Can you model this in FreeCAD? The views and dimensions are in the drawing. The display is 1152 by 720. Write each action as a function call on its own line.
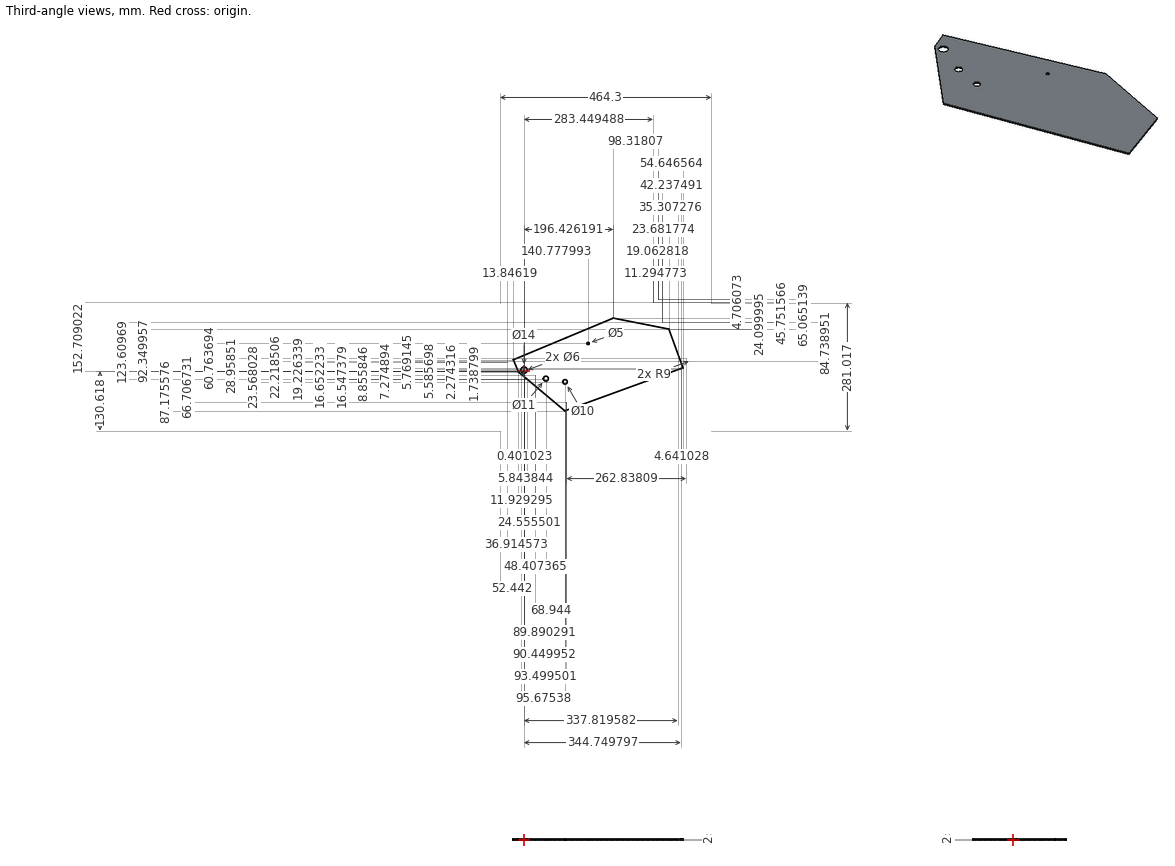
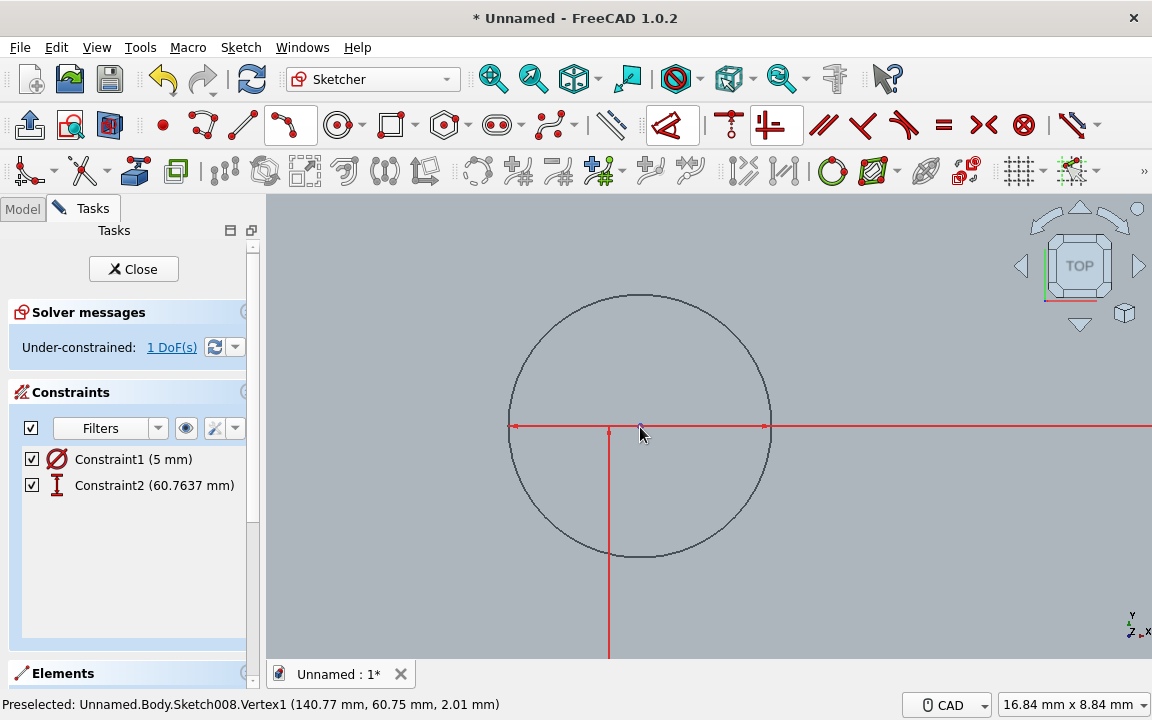
click(640, 426)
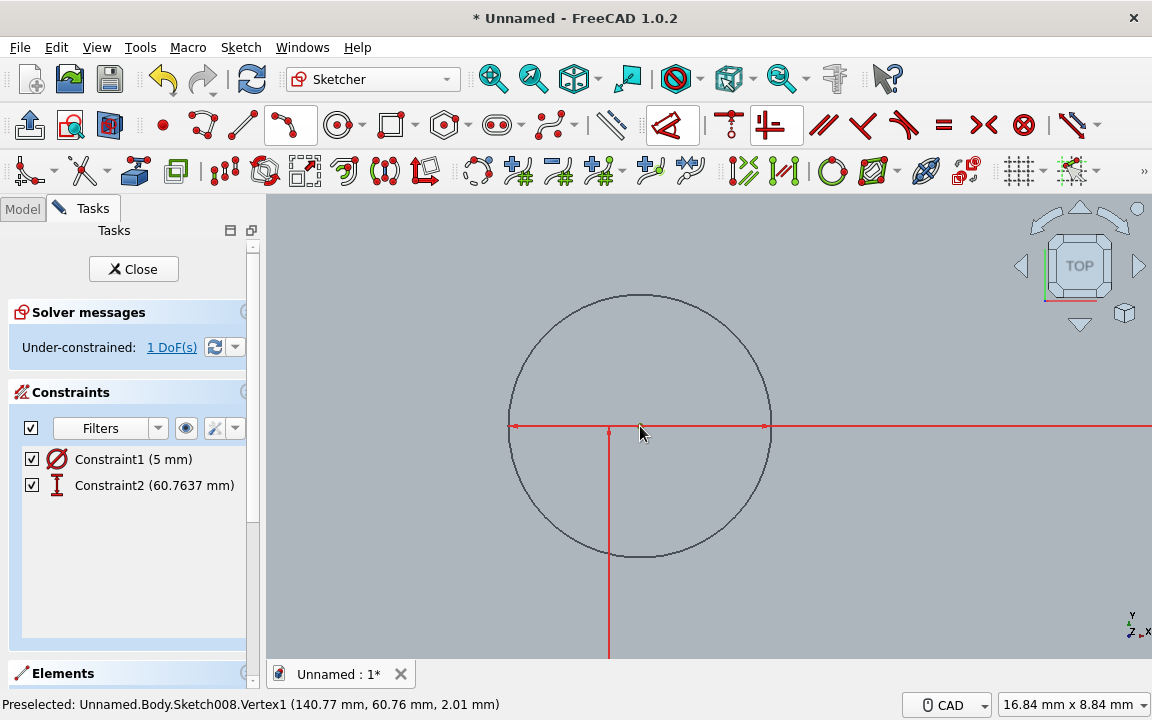
click(694, 126)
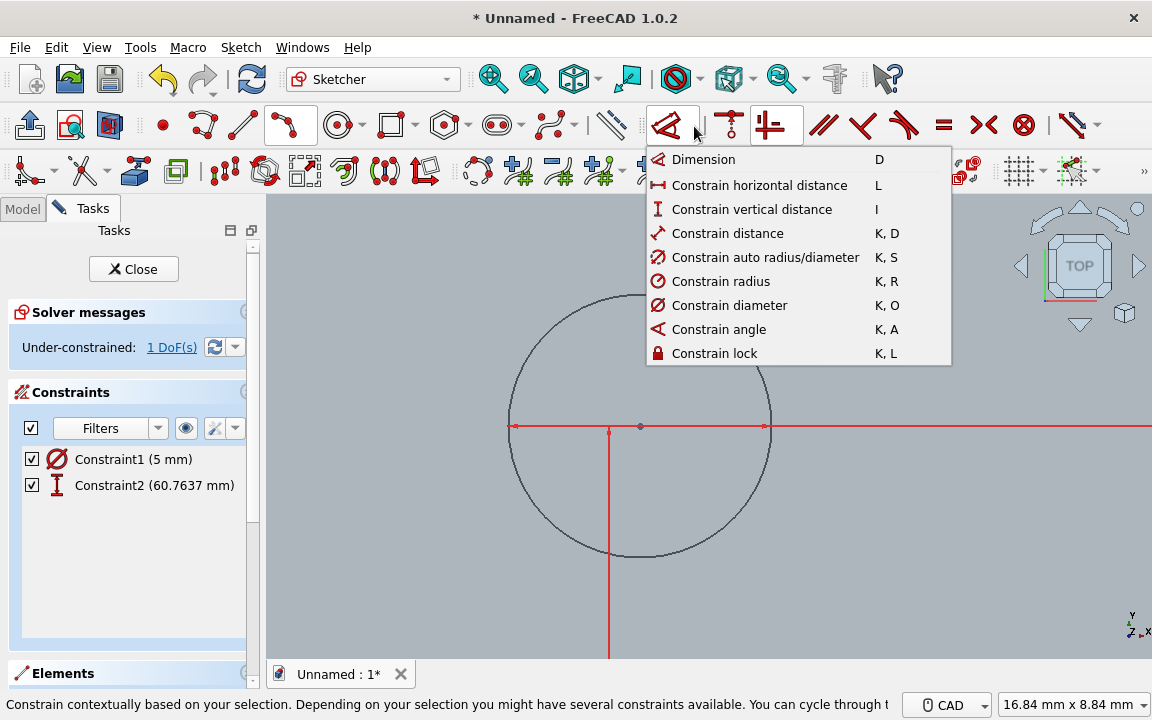
click(799, 185)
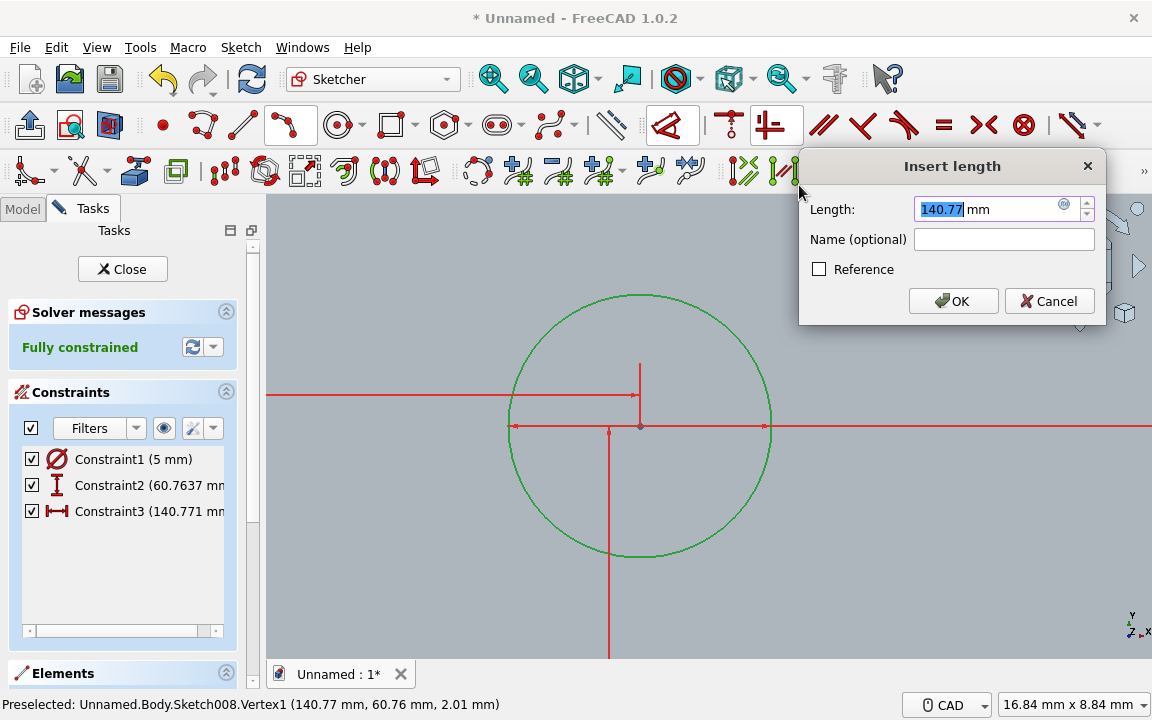
text(140.777993)
key(Return)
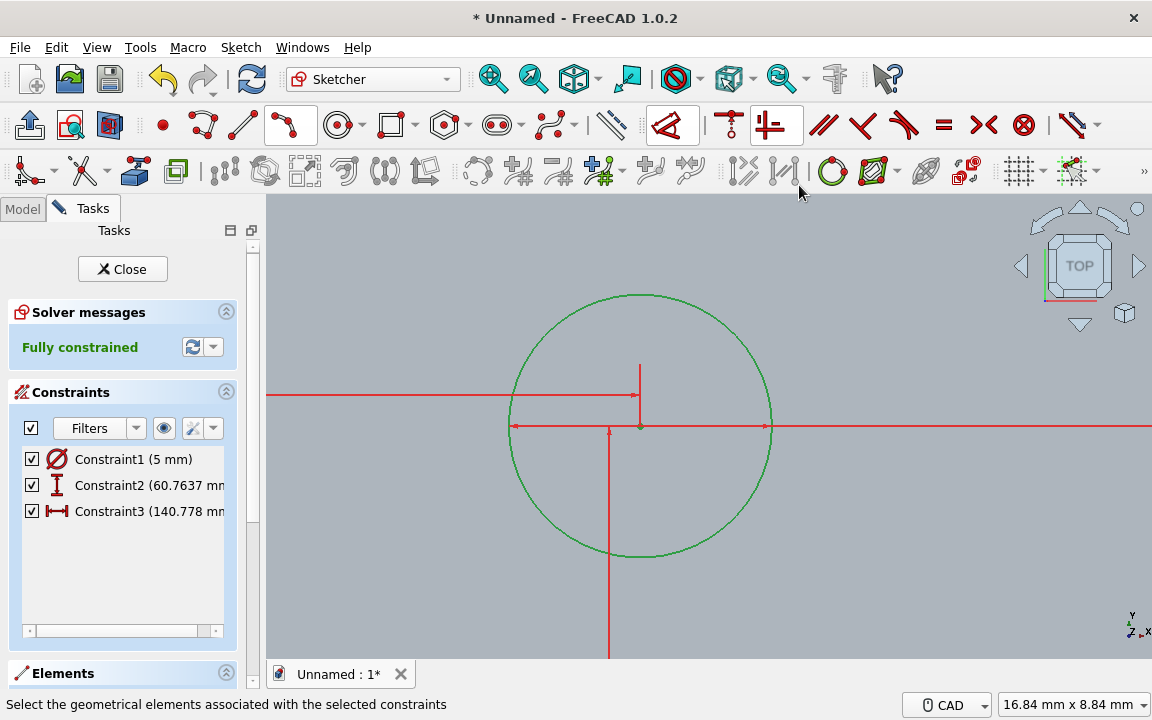
click(123, 269)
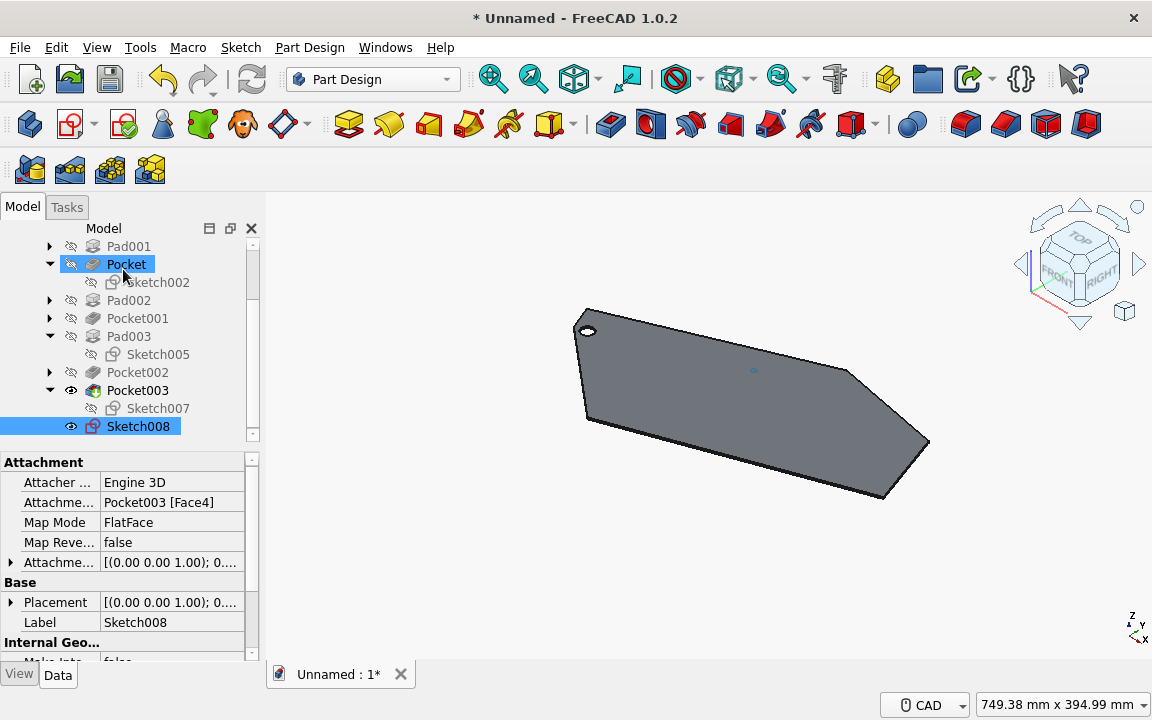
click(612, 124)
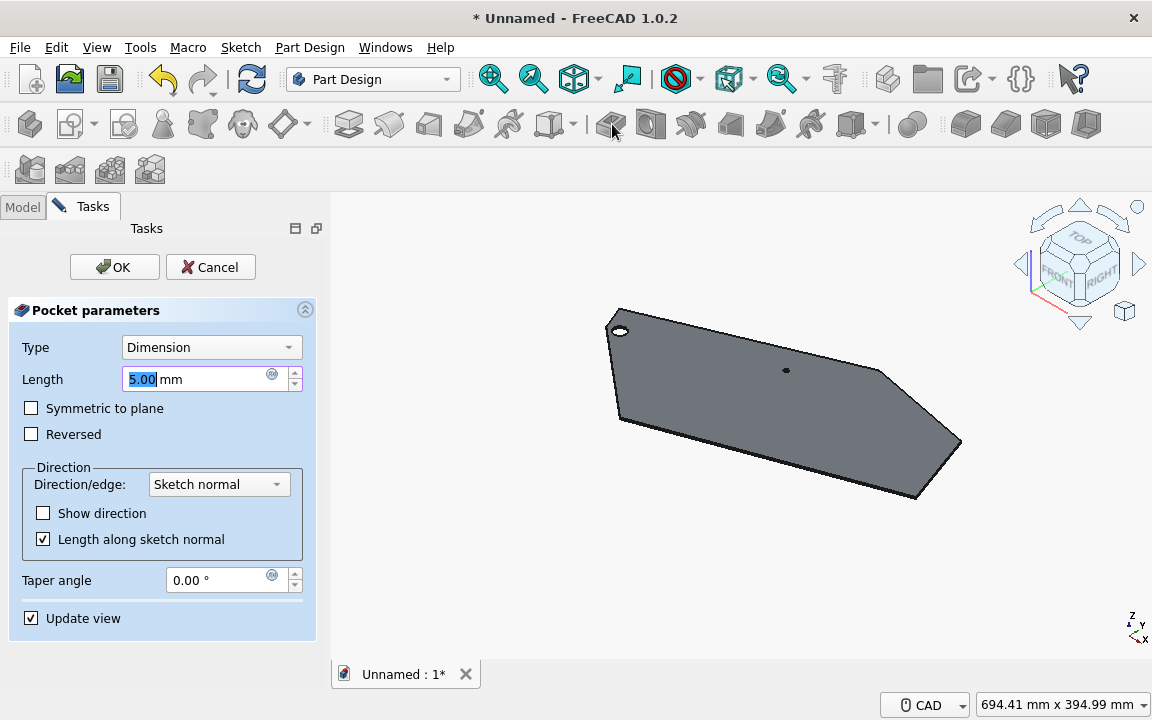
click(212, 348)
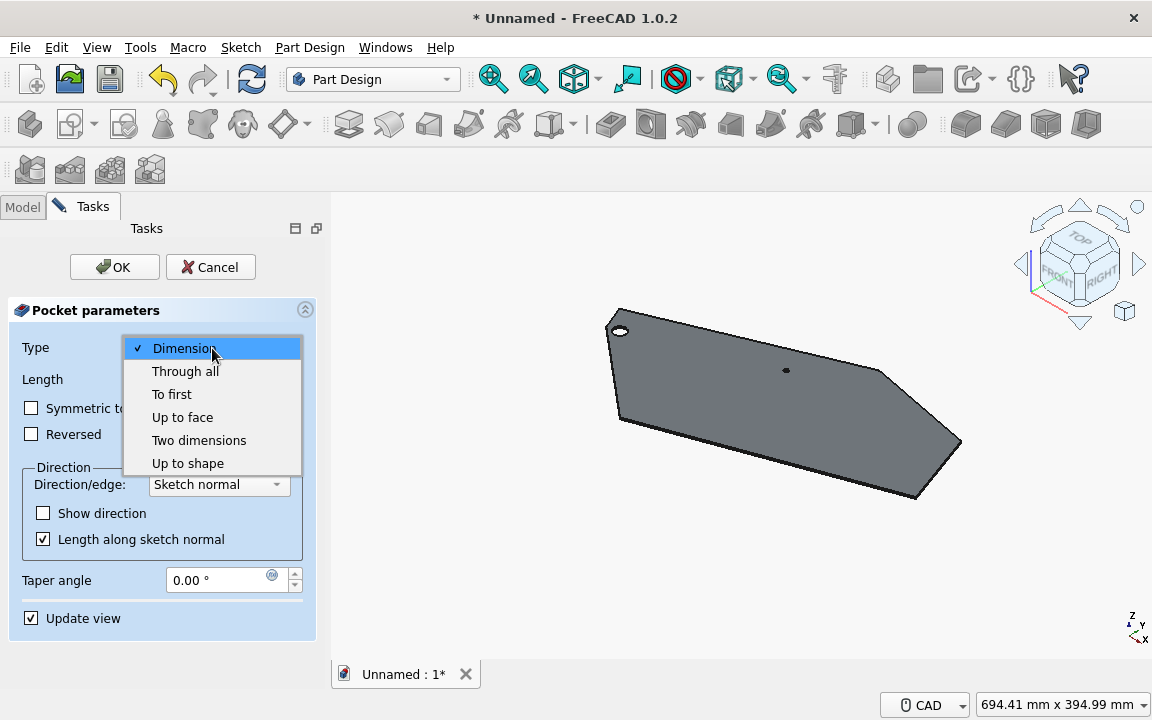
click(212, 372)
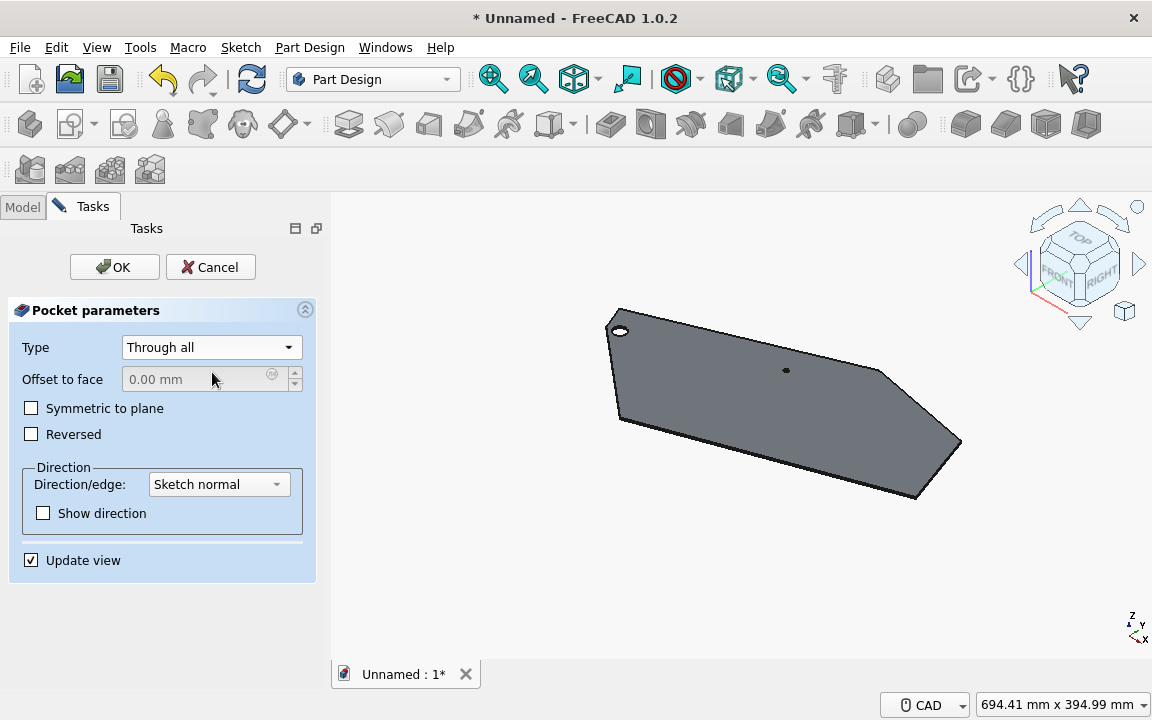
click(115, 267)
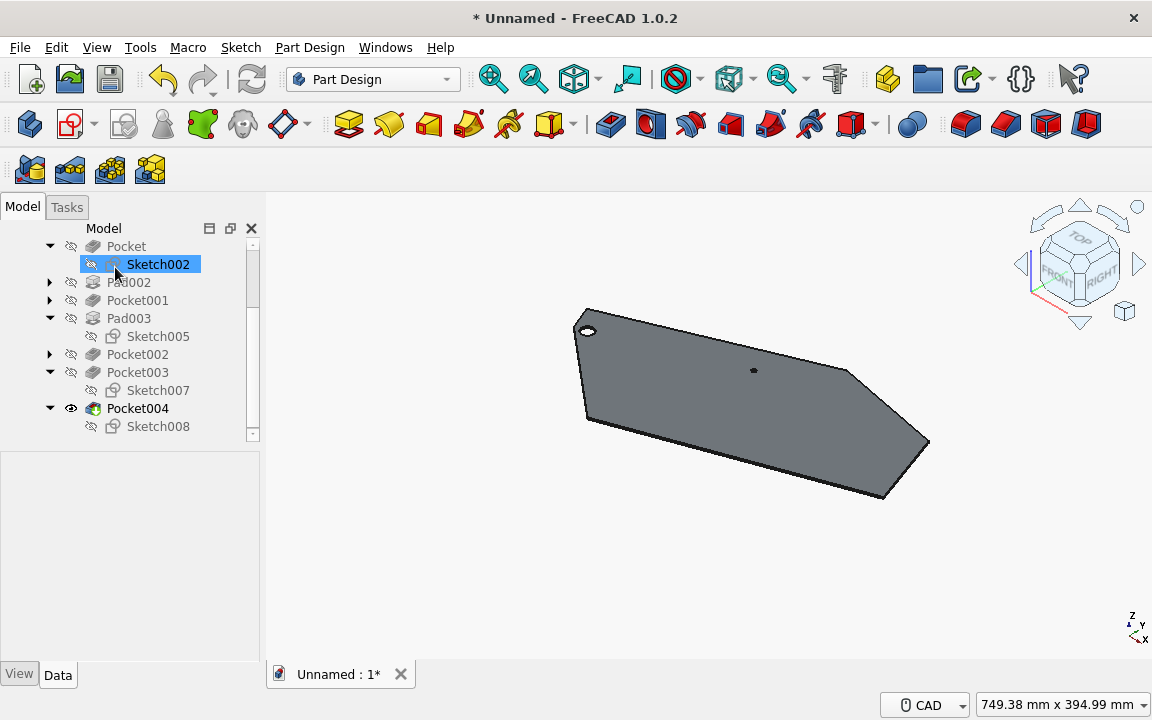
key(5)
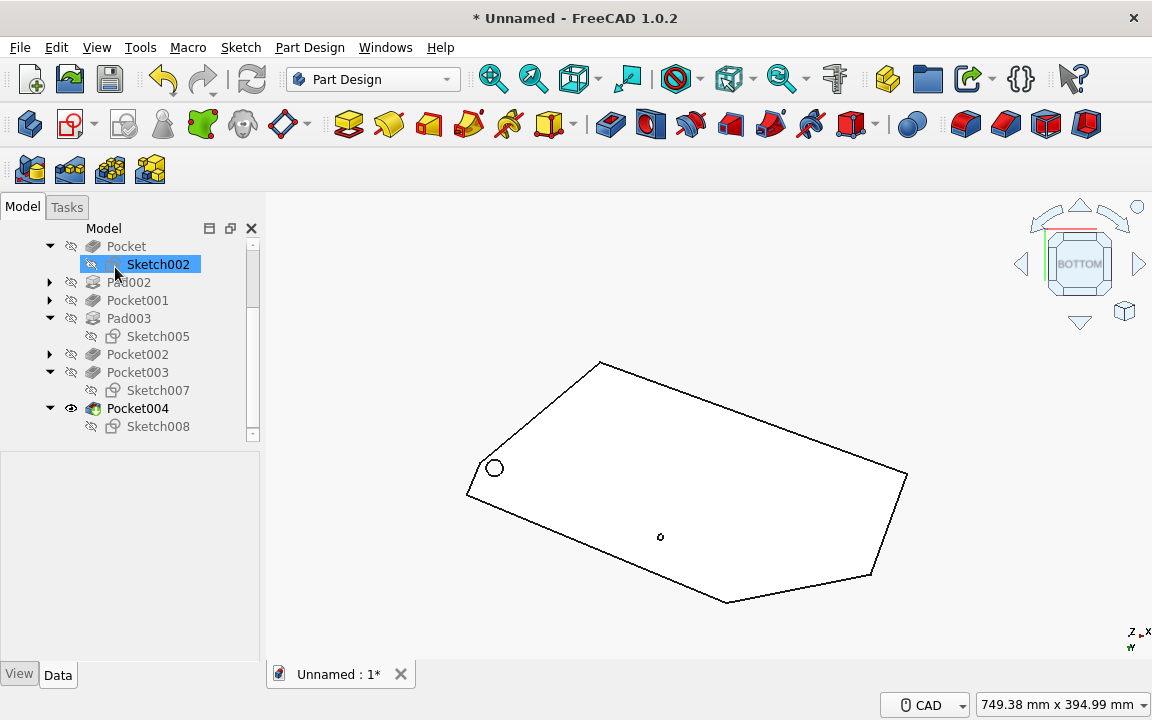
click(750, 516)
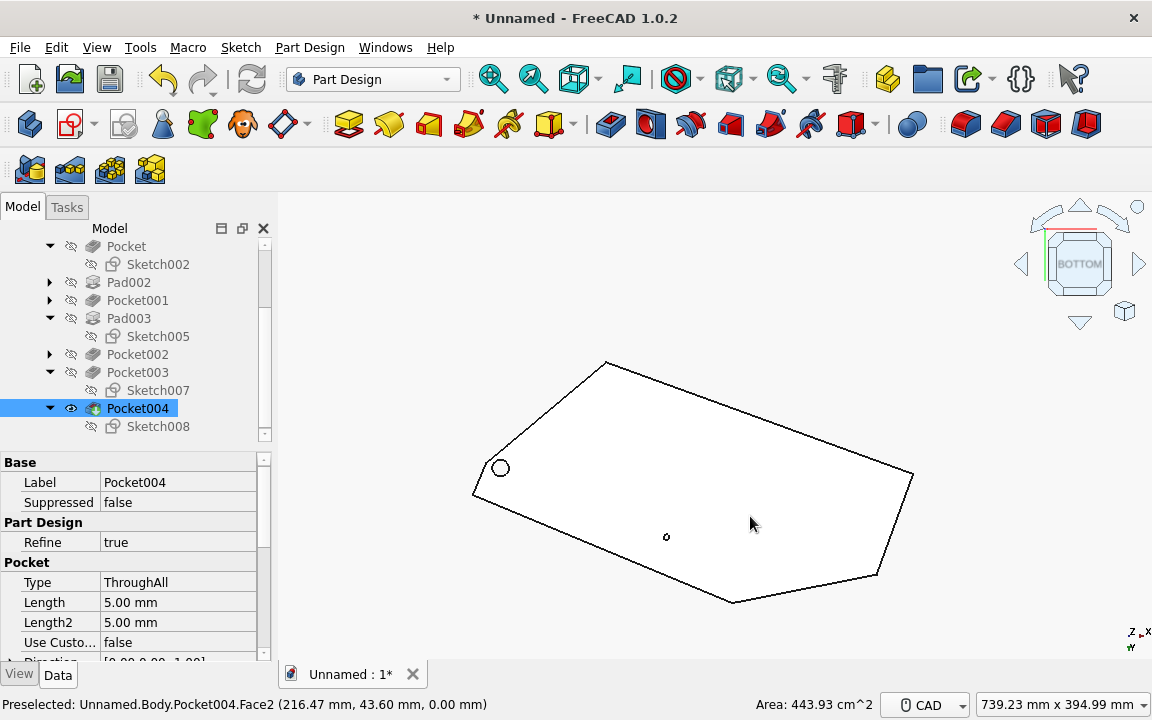
click(70, 124)